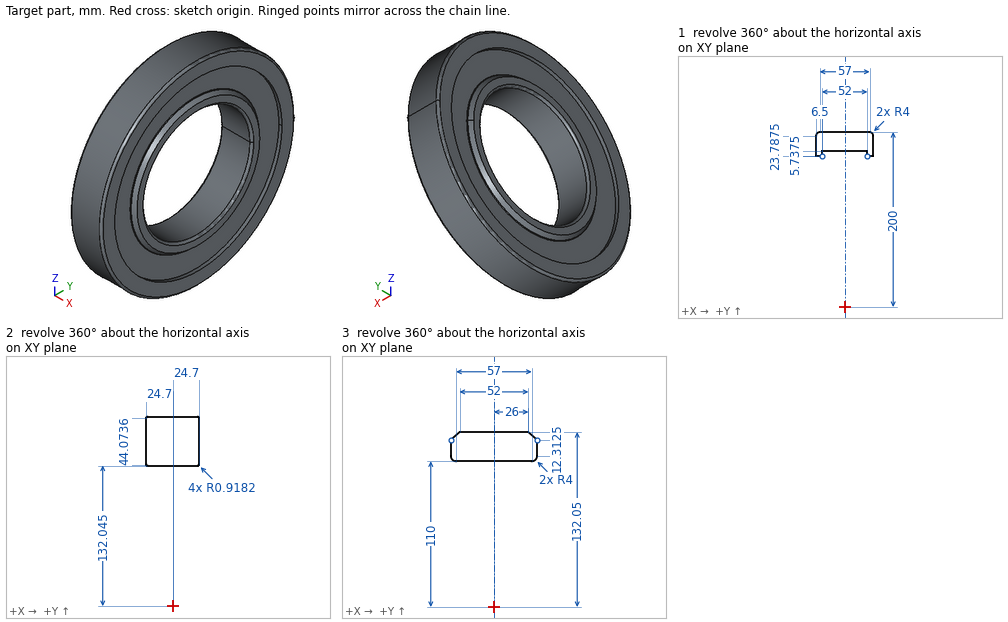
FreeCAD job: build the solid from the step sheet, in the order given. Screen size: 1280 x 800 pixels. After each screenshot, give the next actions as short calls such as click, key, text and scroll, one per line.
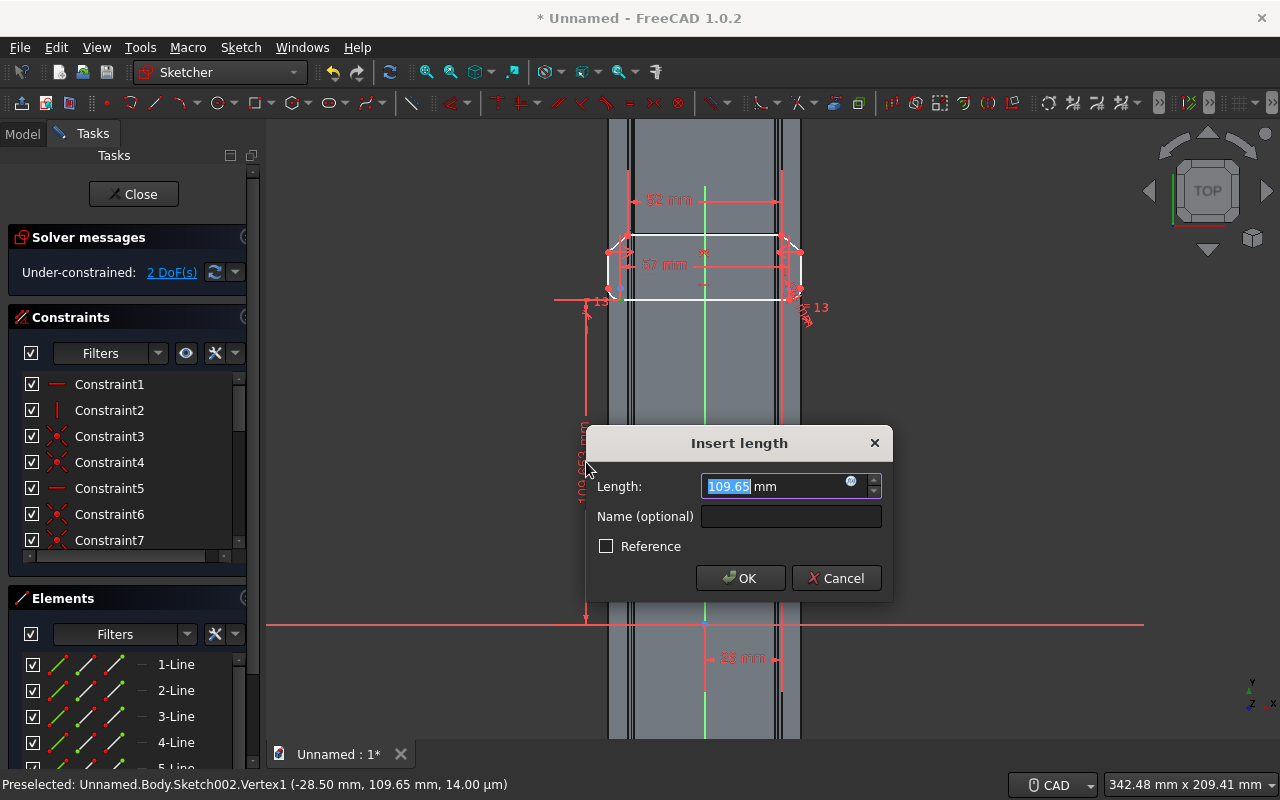
text(110)
key(Return)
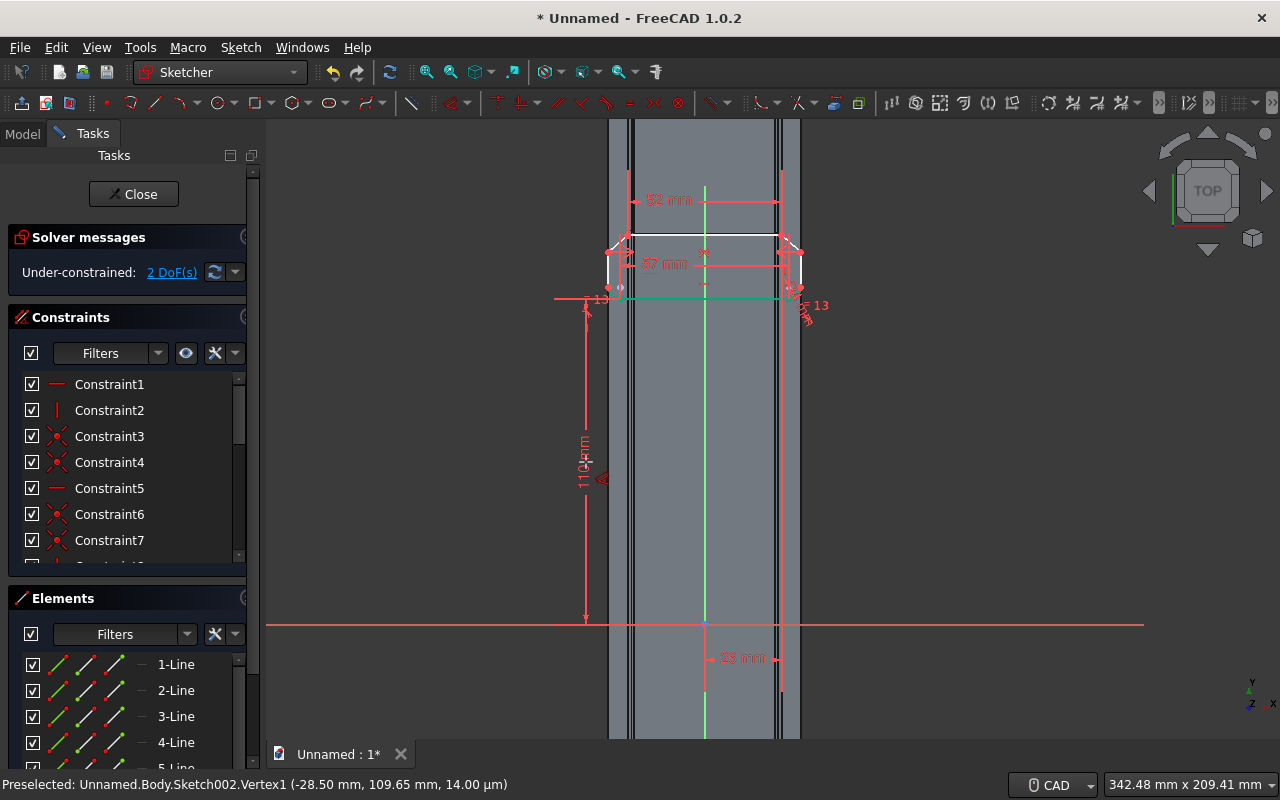
scroll(801, 277, up, 2)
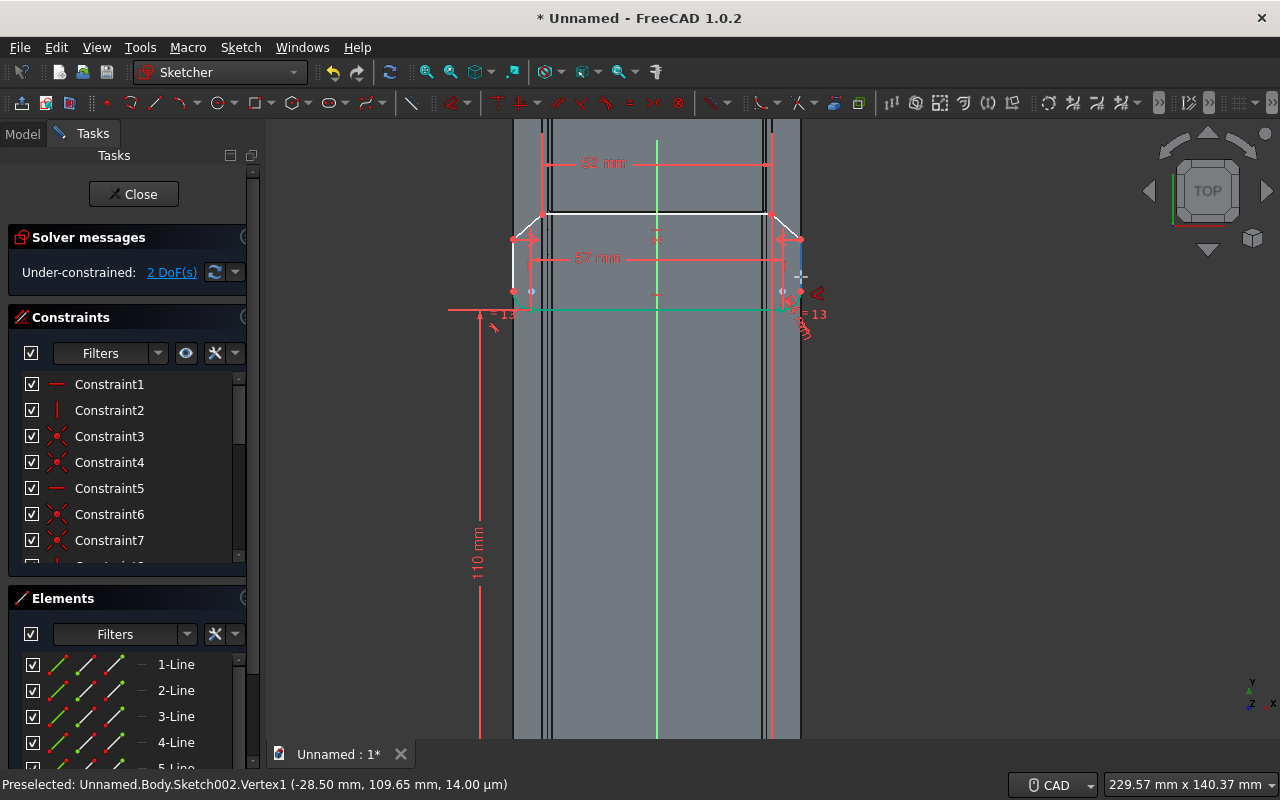
click(801, 276)
click(835, 266)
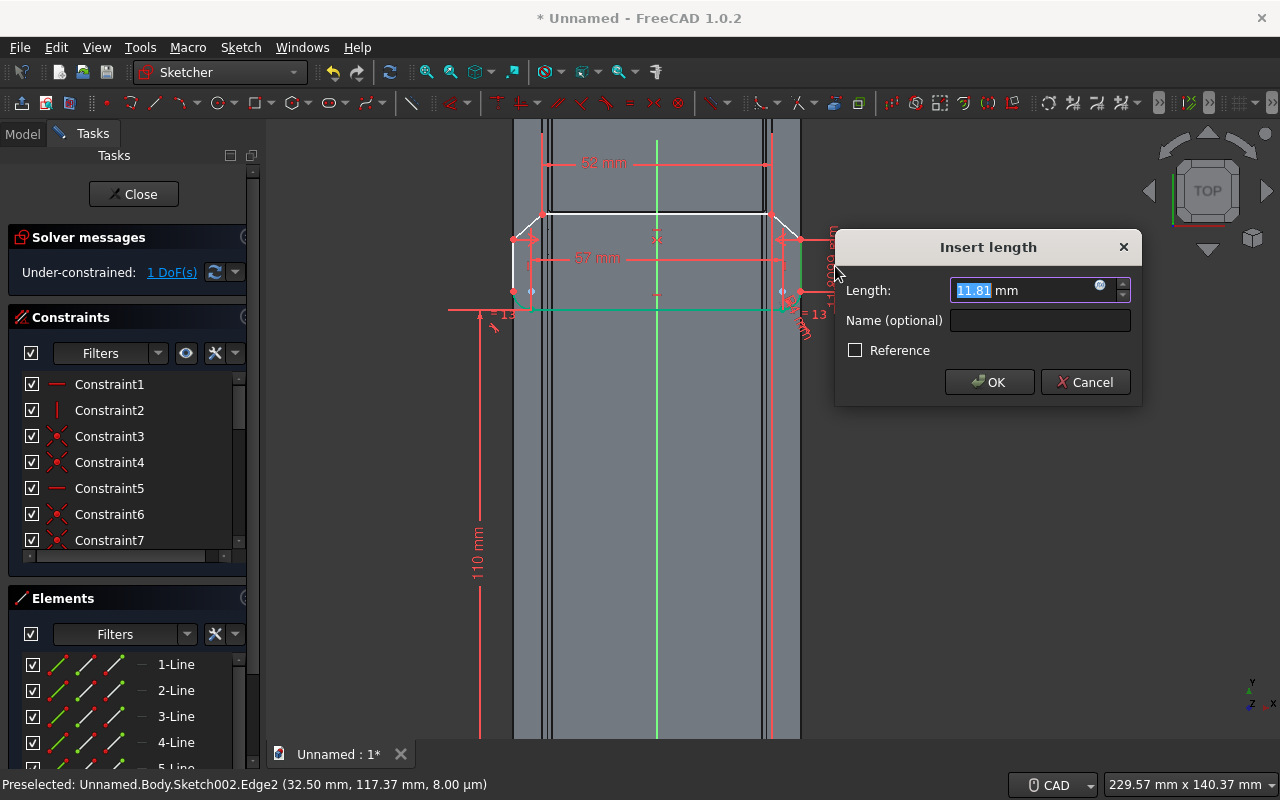
text(12.3125)
key(Return)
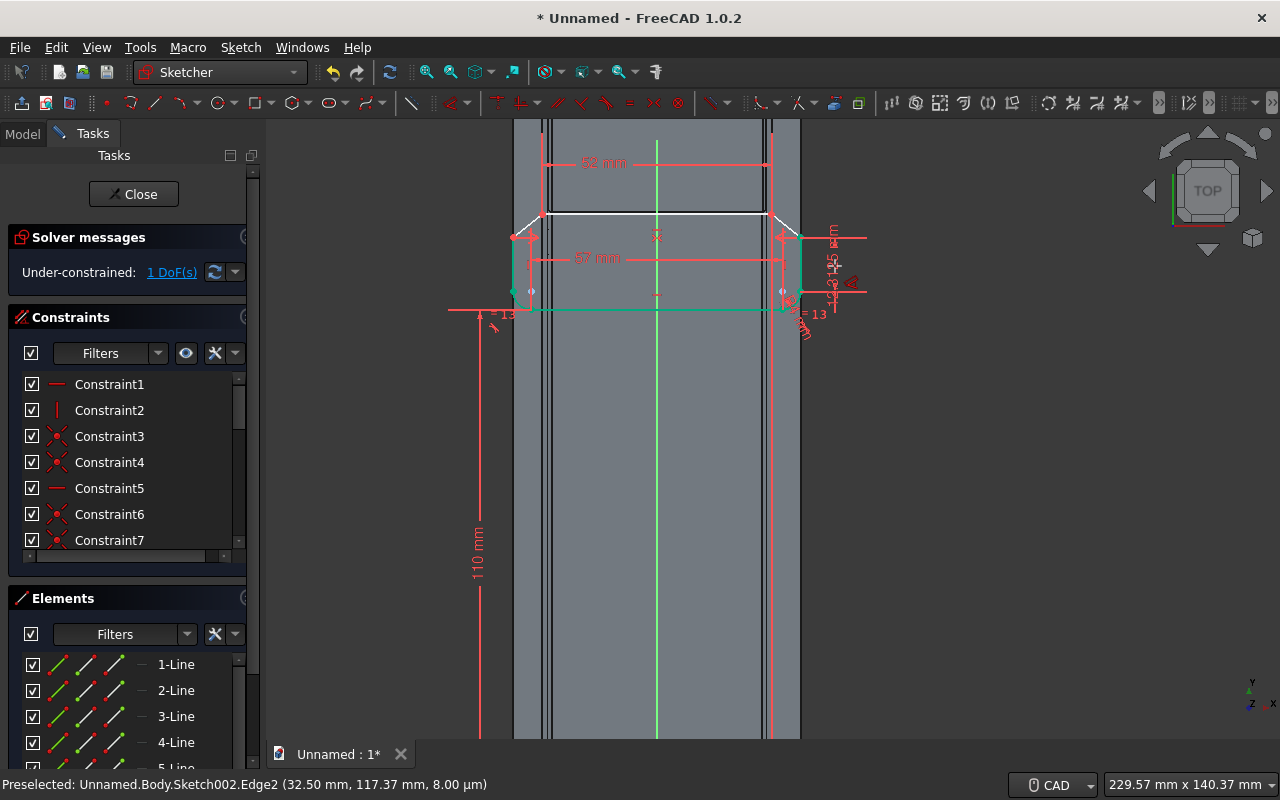
click(772, 214)
click(806, 463)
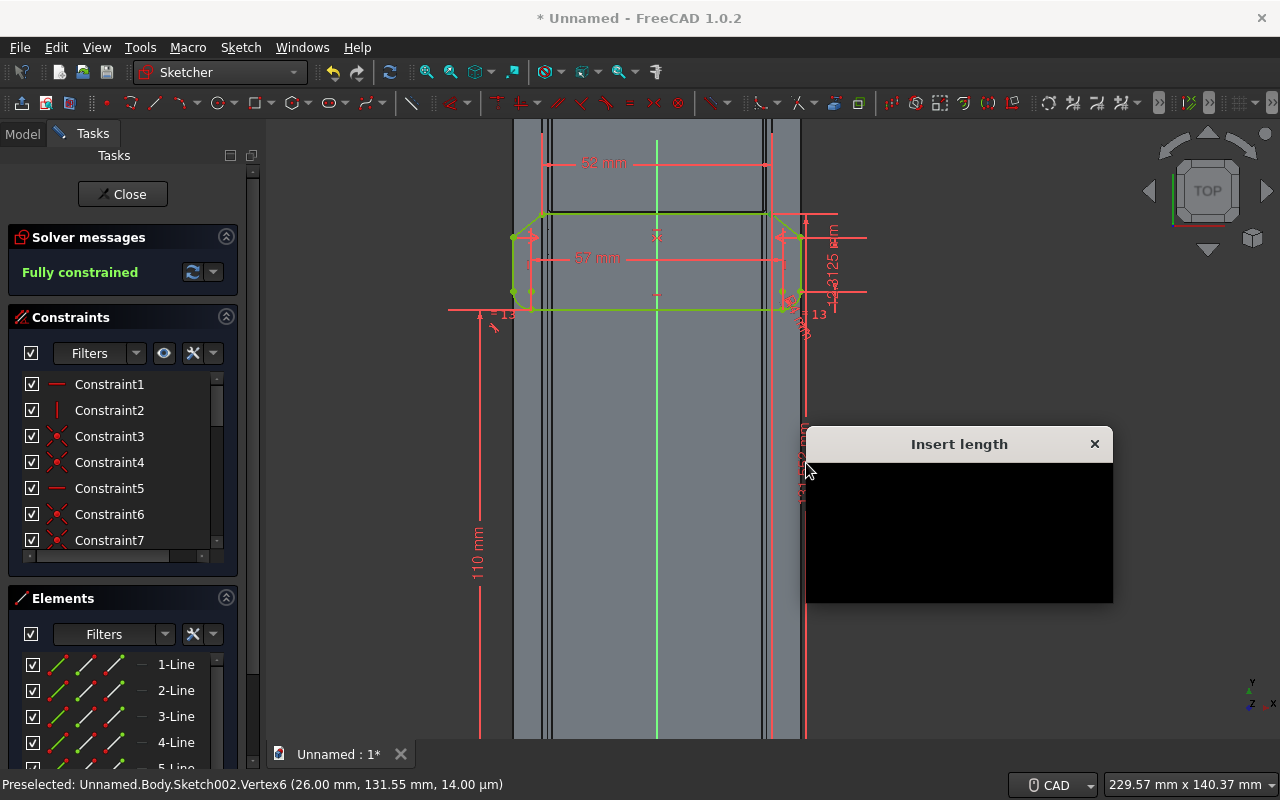
text(132.05)
key(Return)
key(Escape)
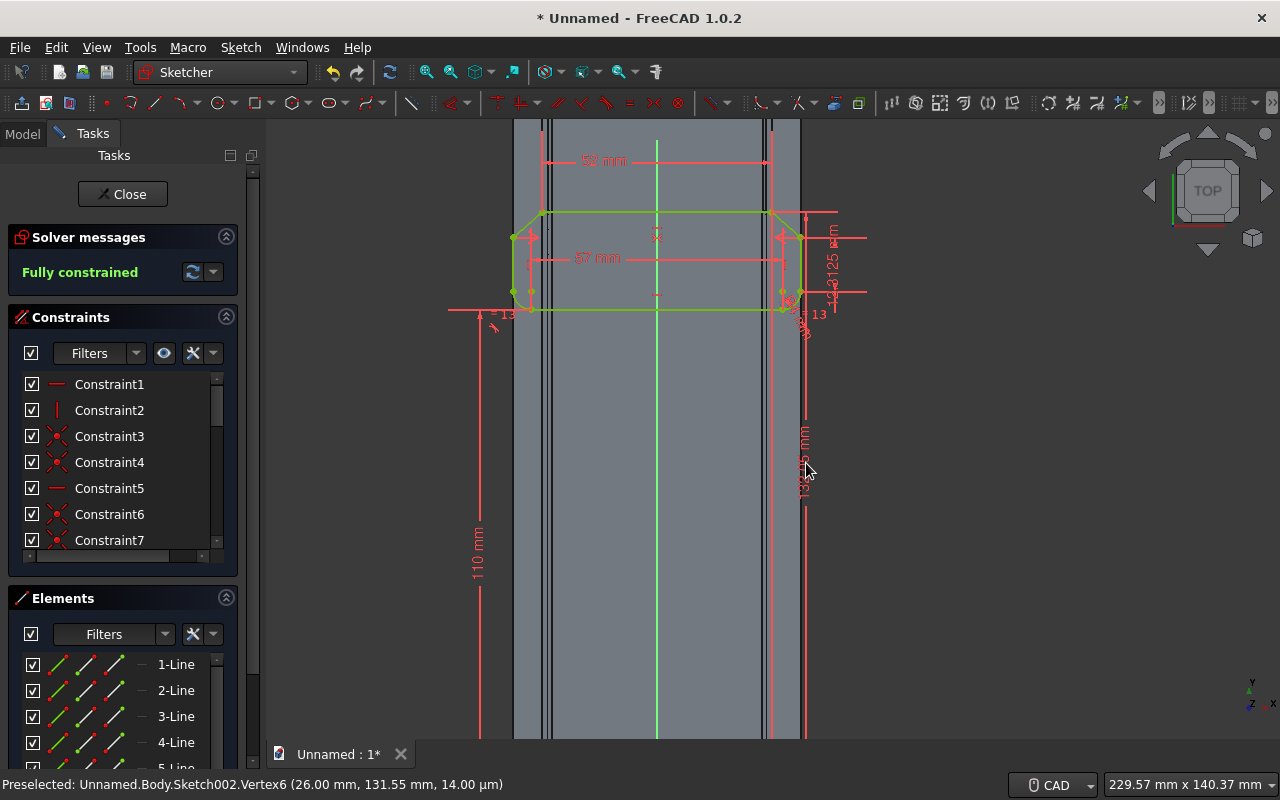
click(123, 194)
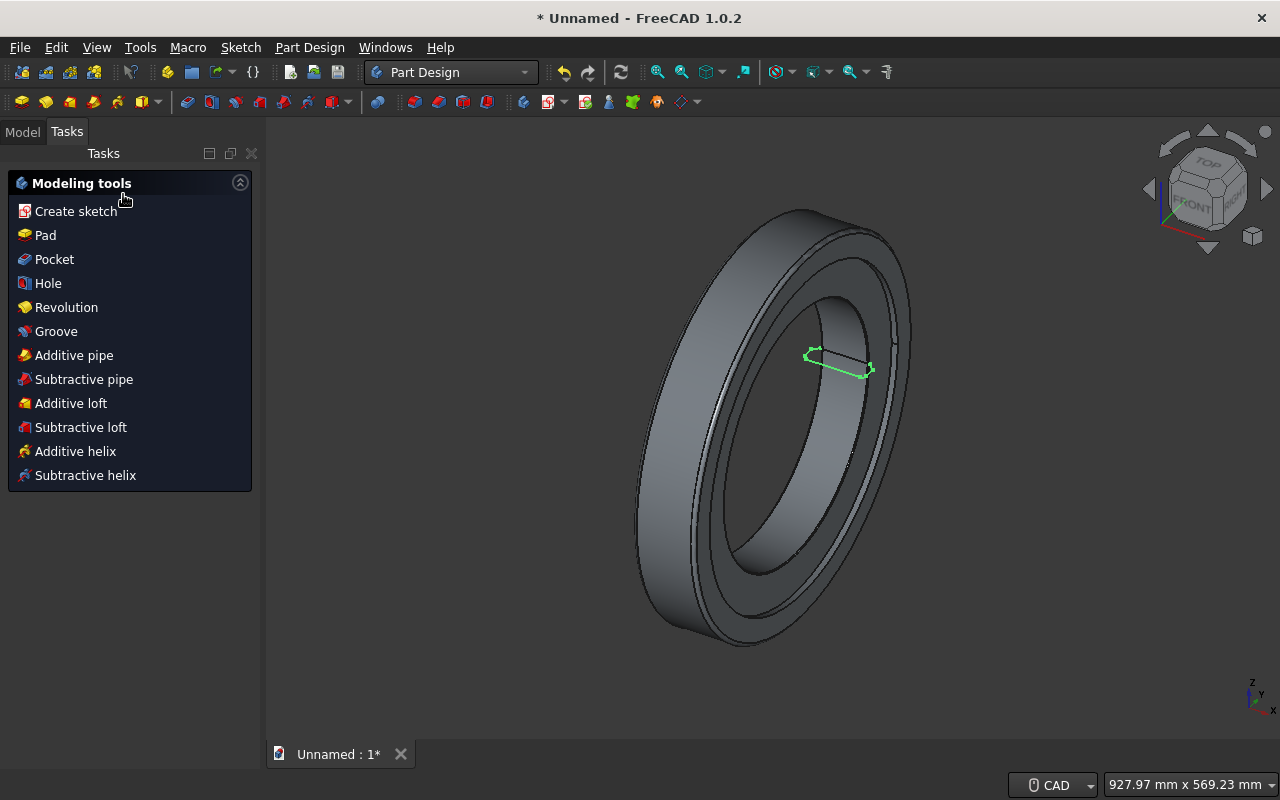
click(46, 102)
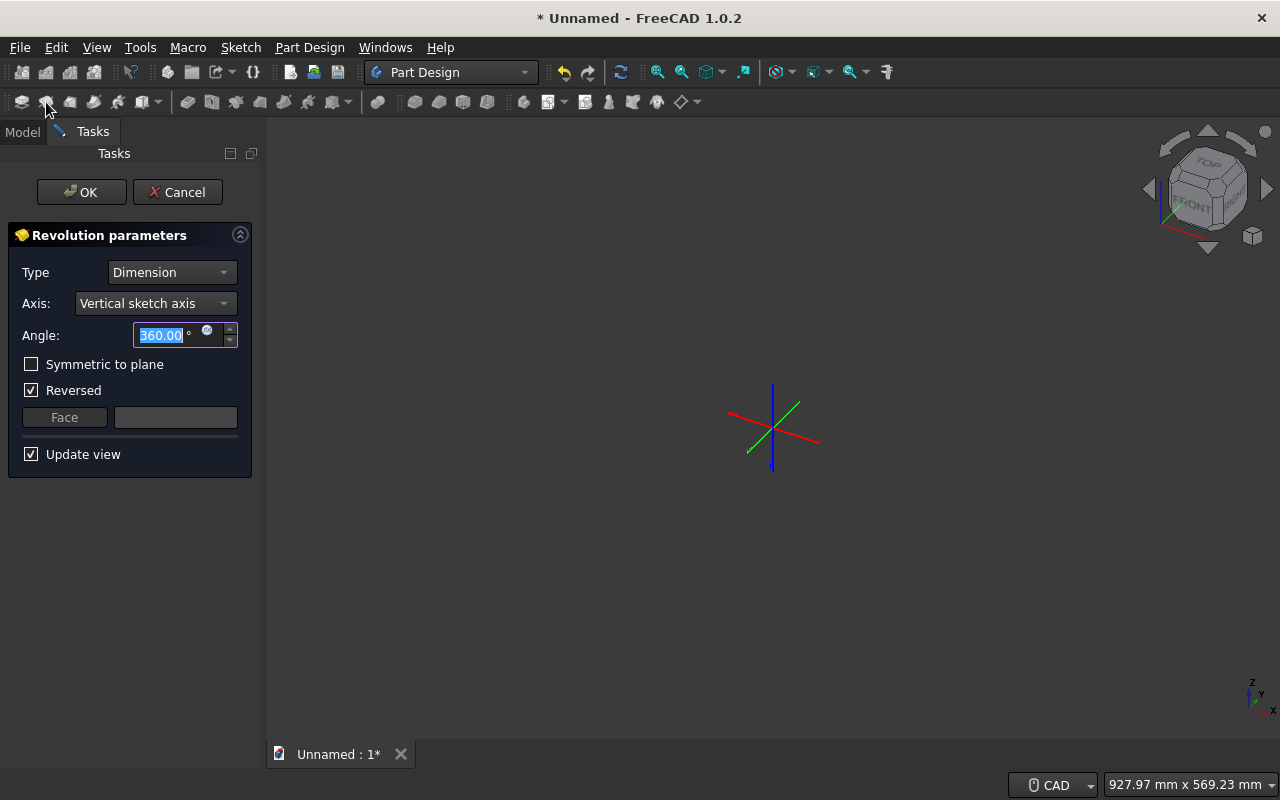
click(156, 304)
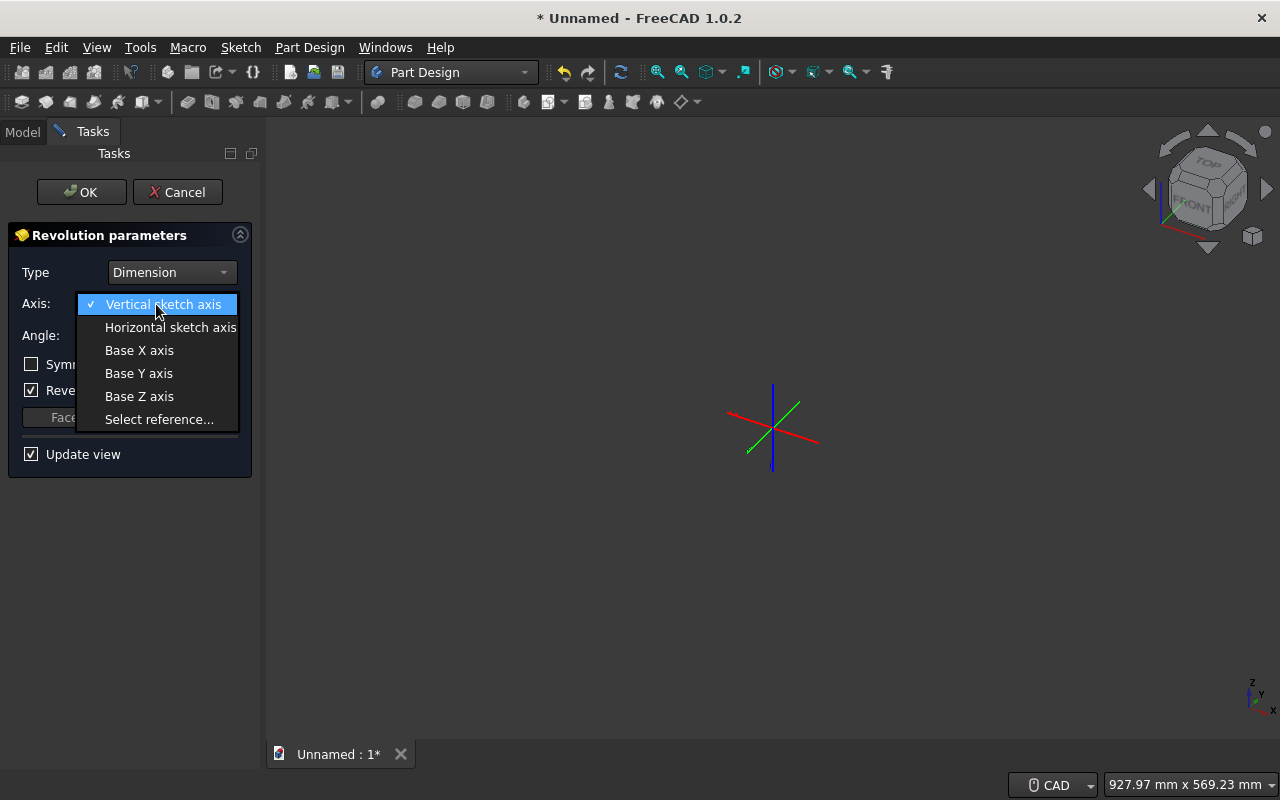
click(156, 328)